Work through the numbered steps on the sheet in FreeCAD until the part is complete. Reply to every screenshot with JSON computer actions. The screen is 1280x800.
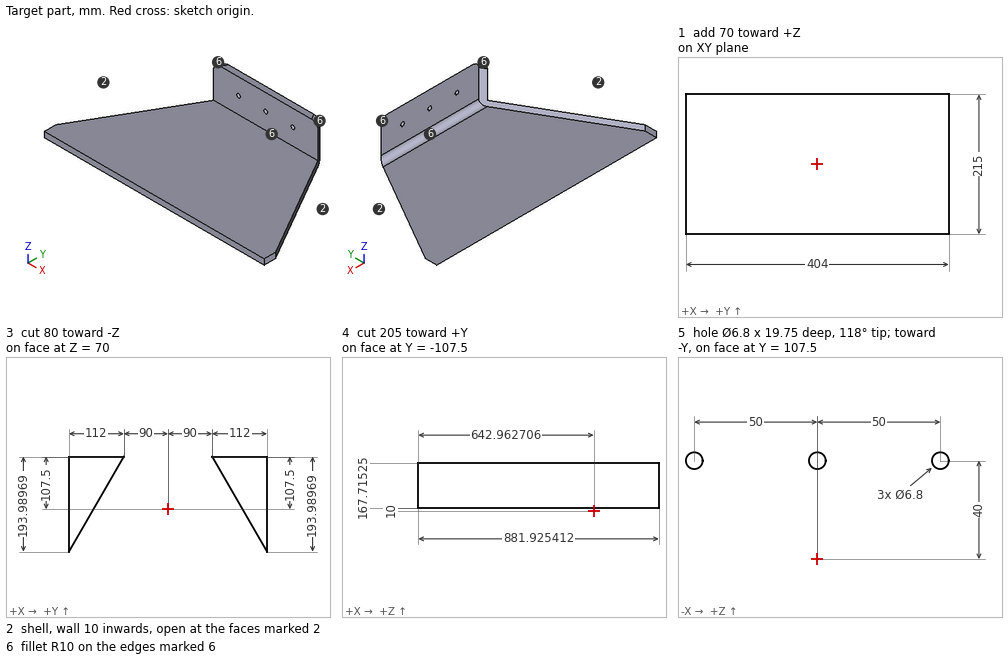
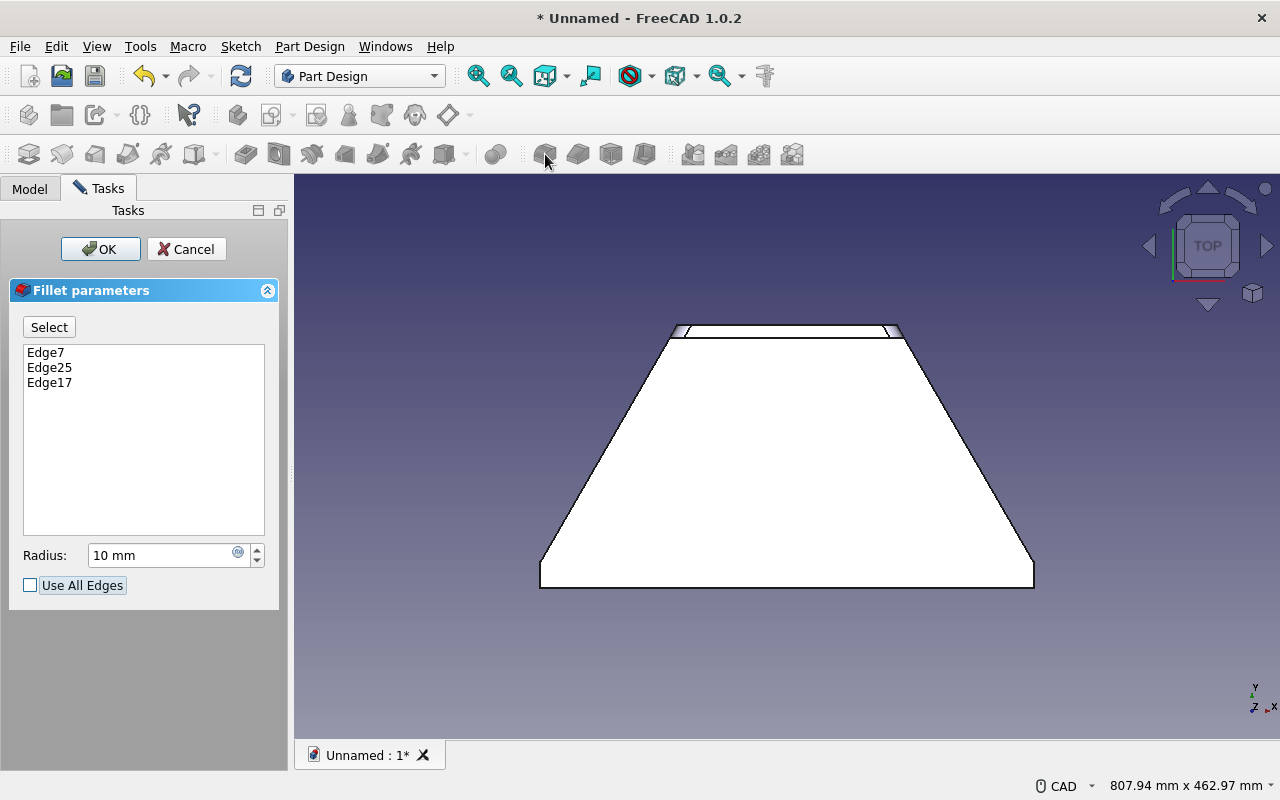
{"action": "left_click", "coordinate": [101, 249]}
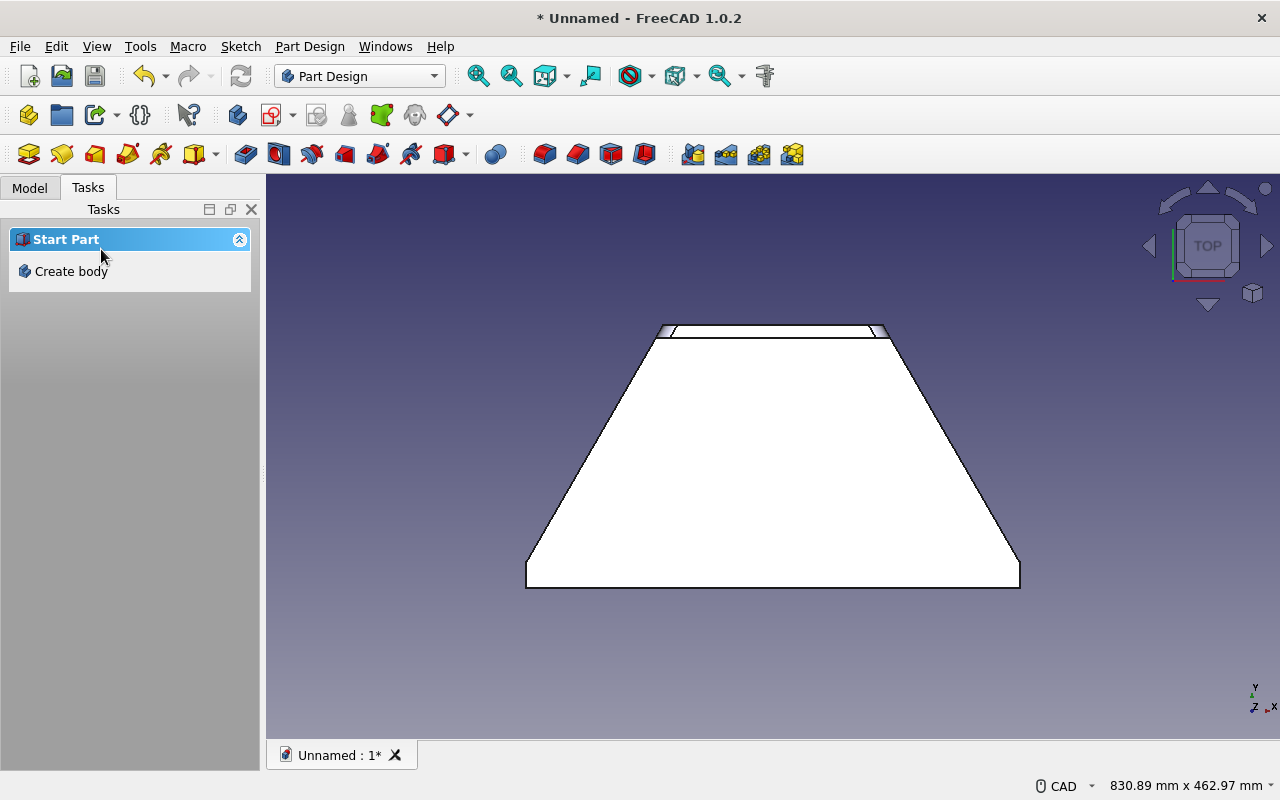
{"action": "key", "text": "0"}